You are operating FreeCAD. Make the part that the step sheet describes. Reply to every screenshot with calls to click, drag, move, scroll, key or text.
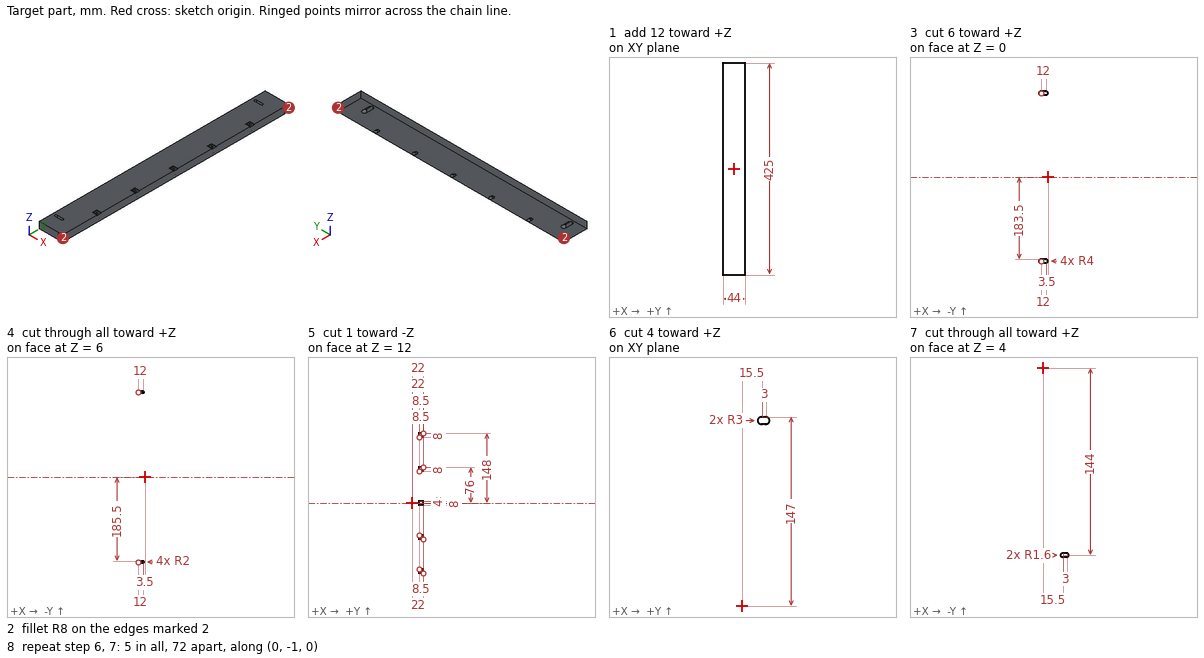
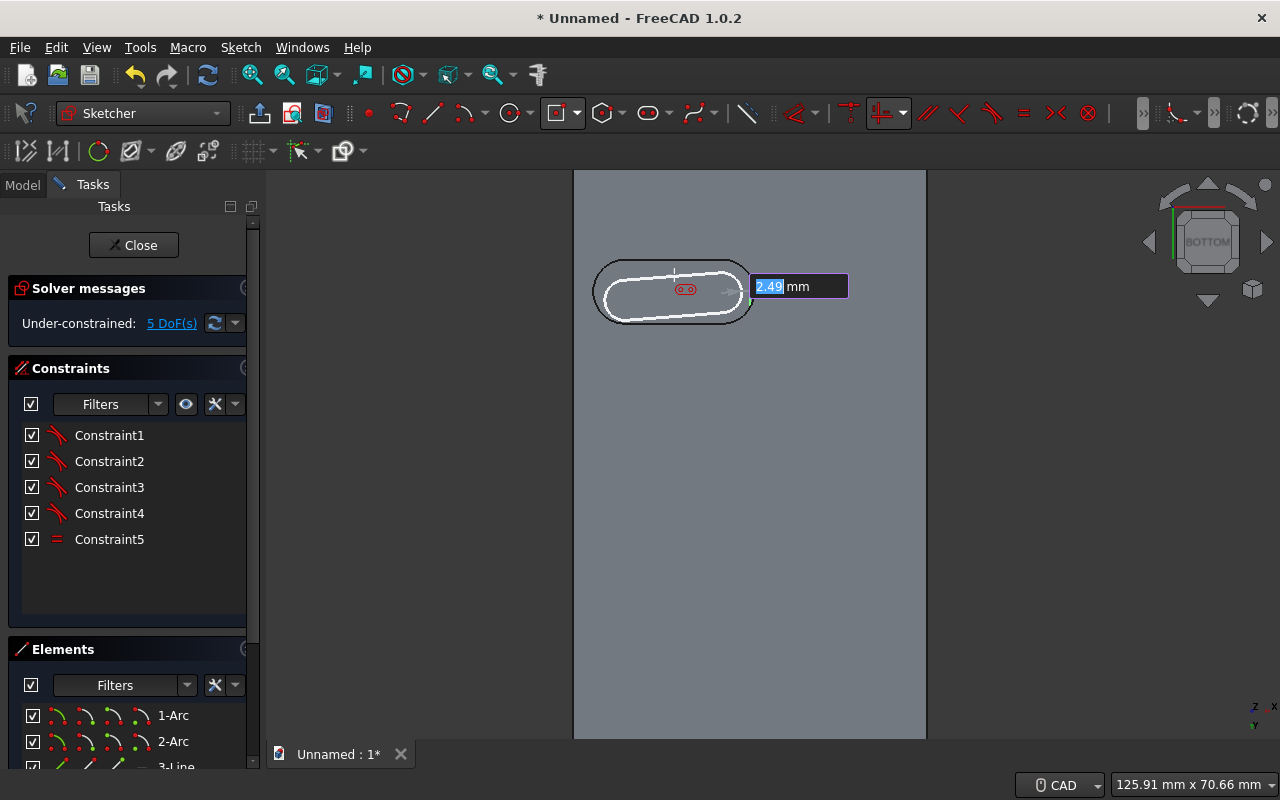
click(674, 276)
key(Escape)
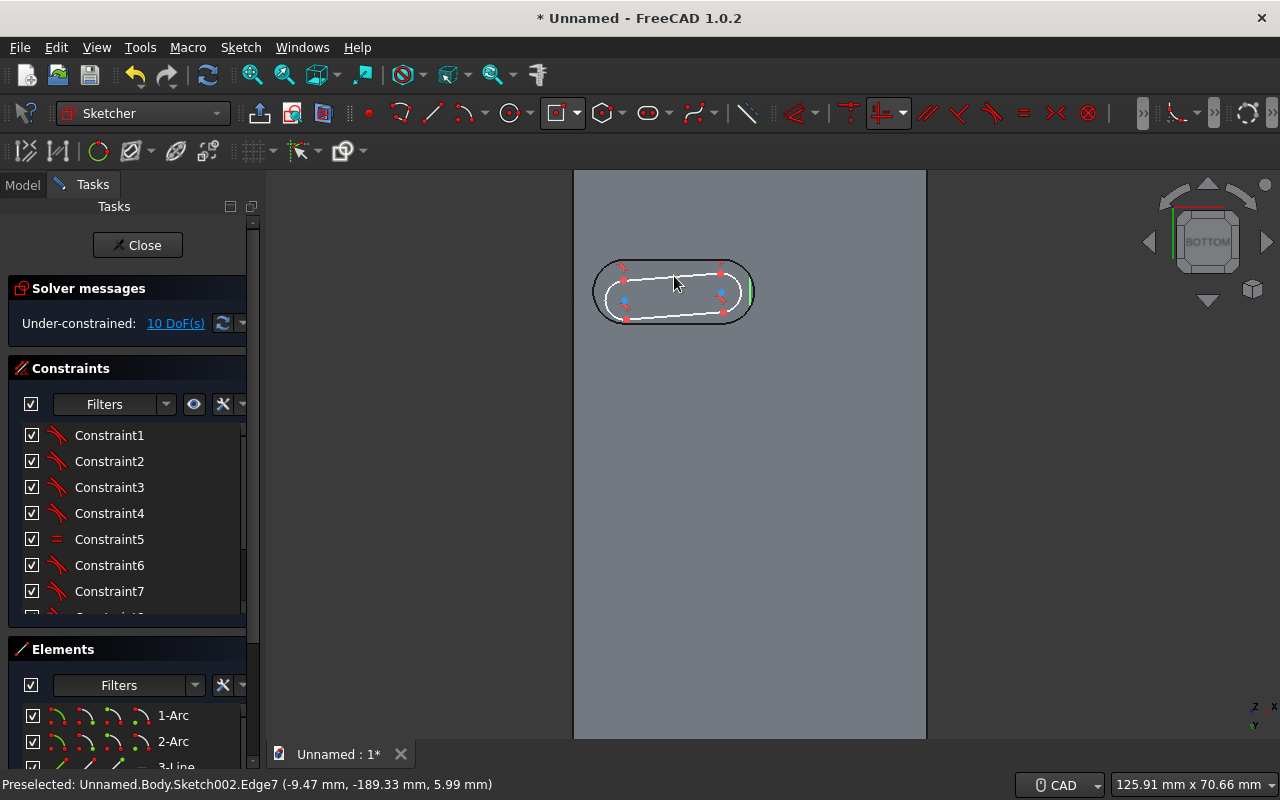
scroll(708, 287, down, 11)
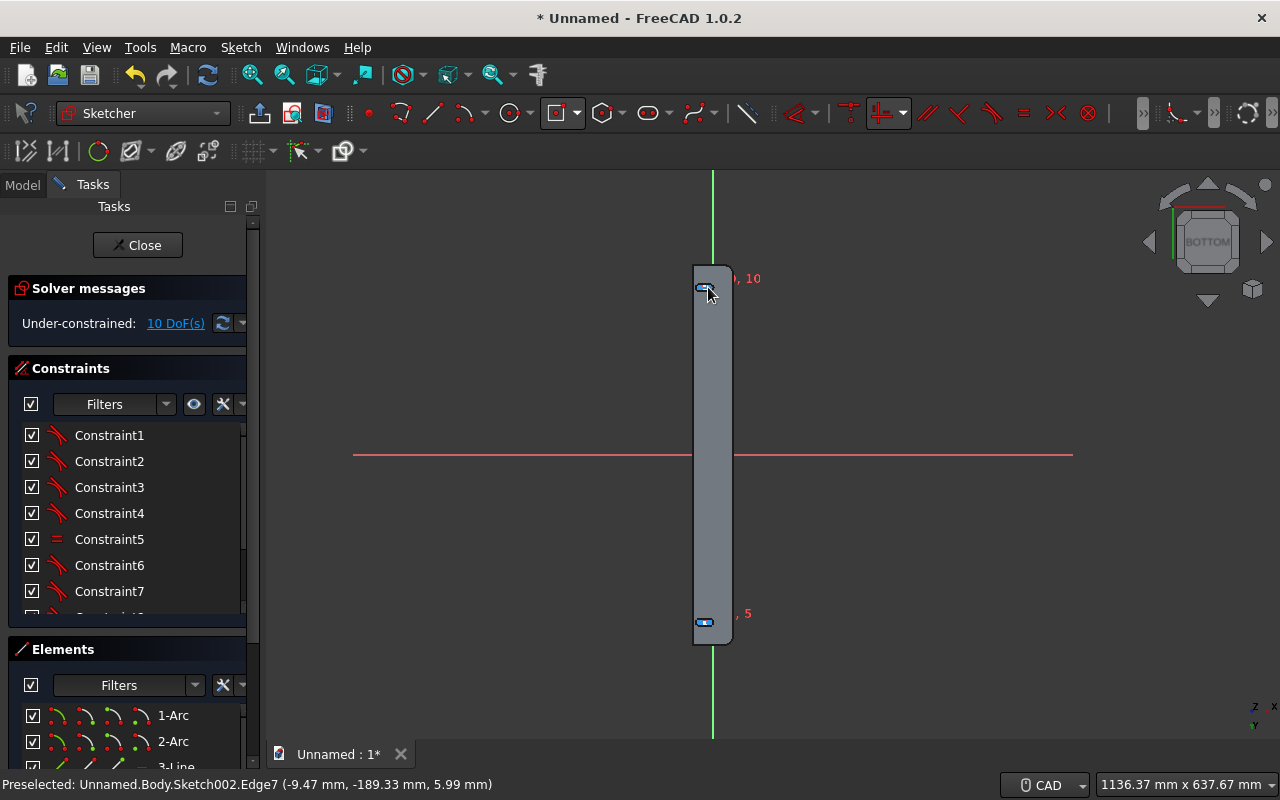
scroll(702, 622, up, 9)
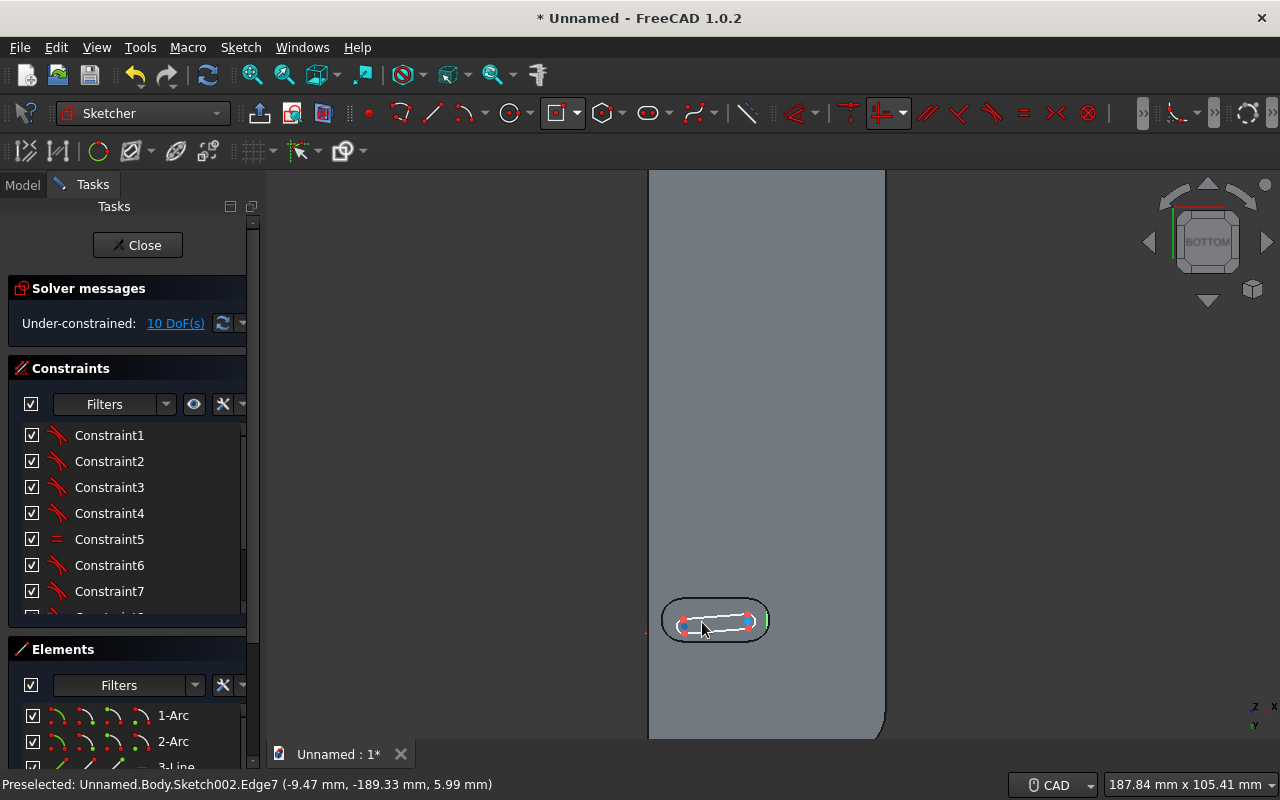
click(703, 618)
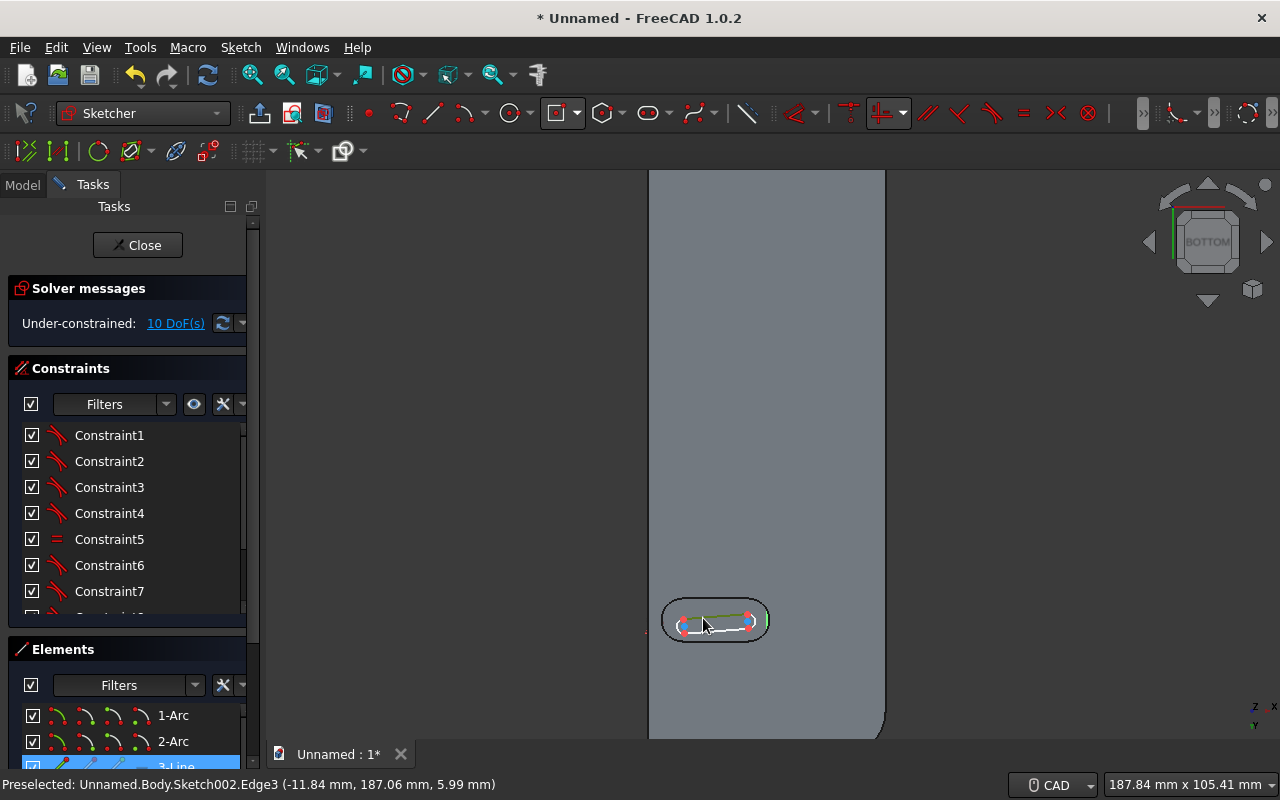
click(906, 114)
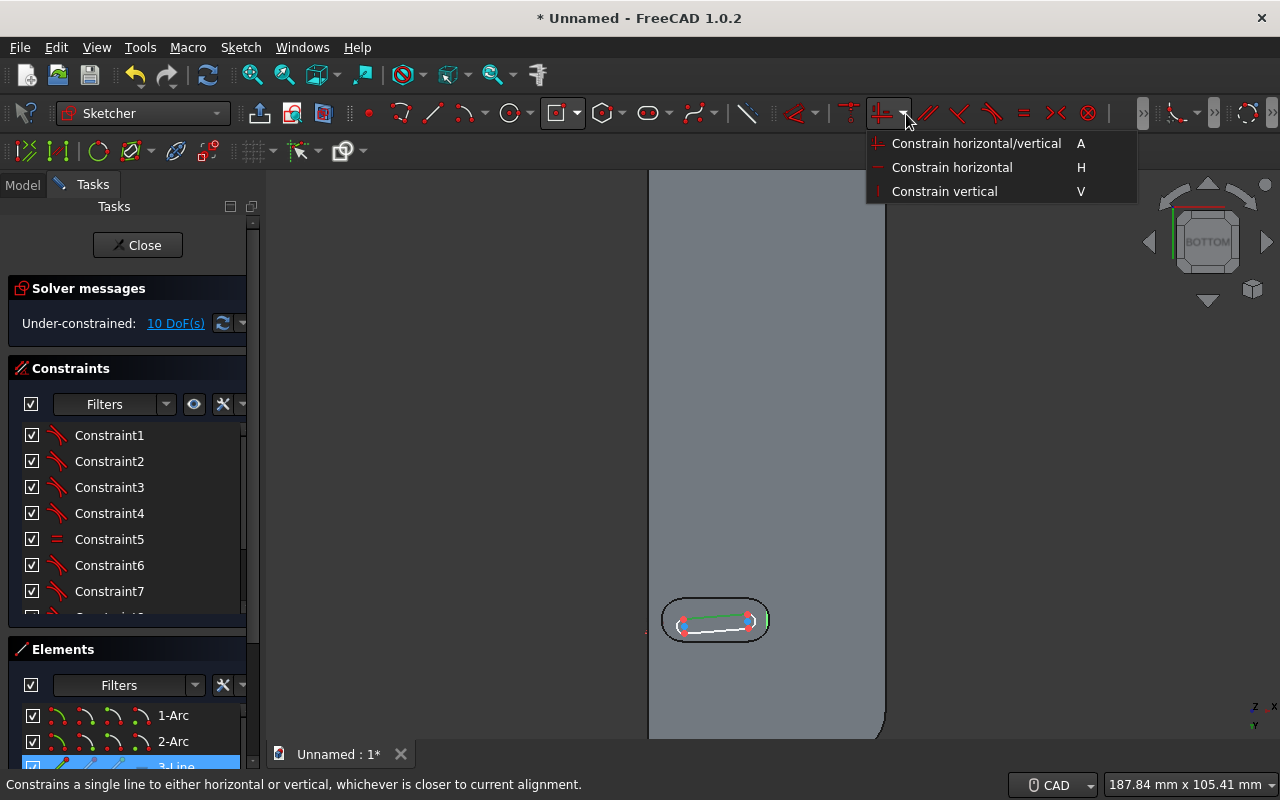
click(1002, 167)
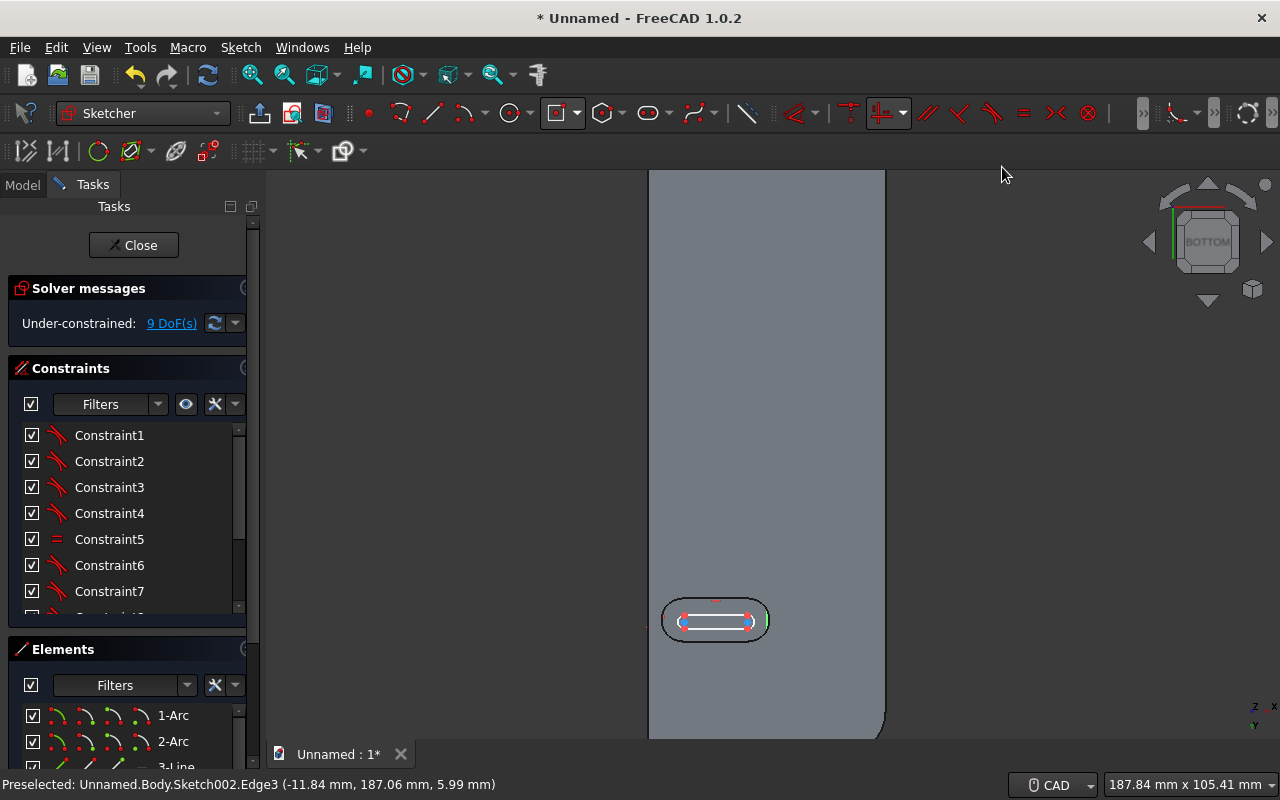
scroll(702, 622, down, 9)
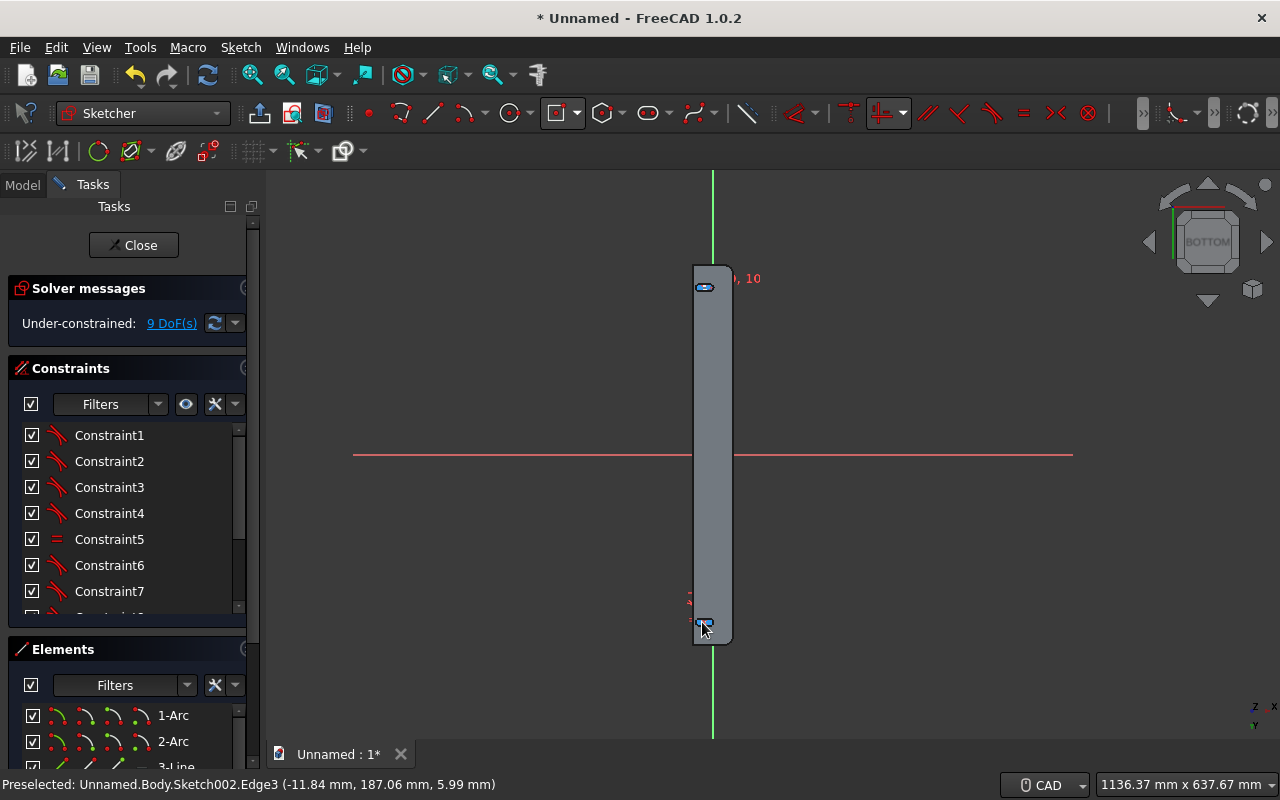
scroll(702, 286, up, 8)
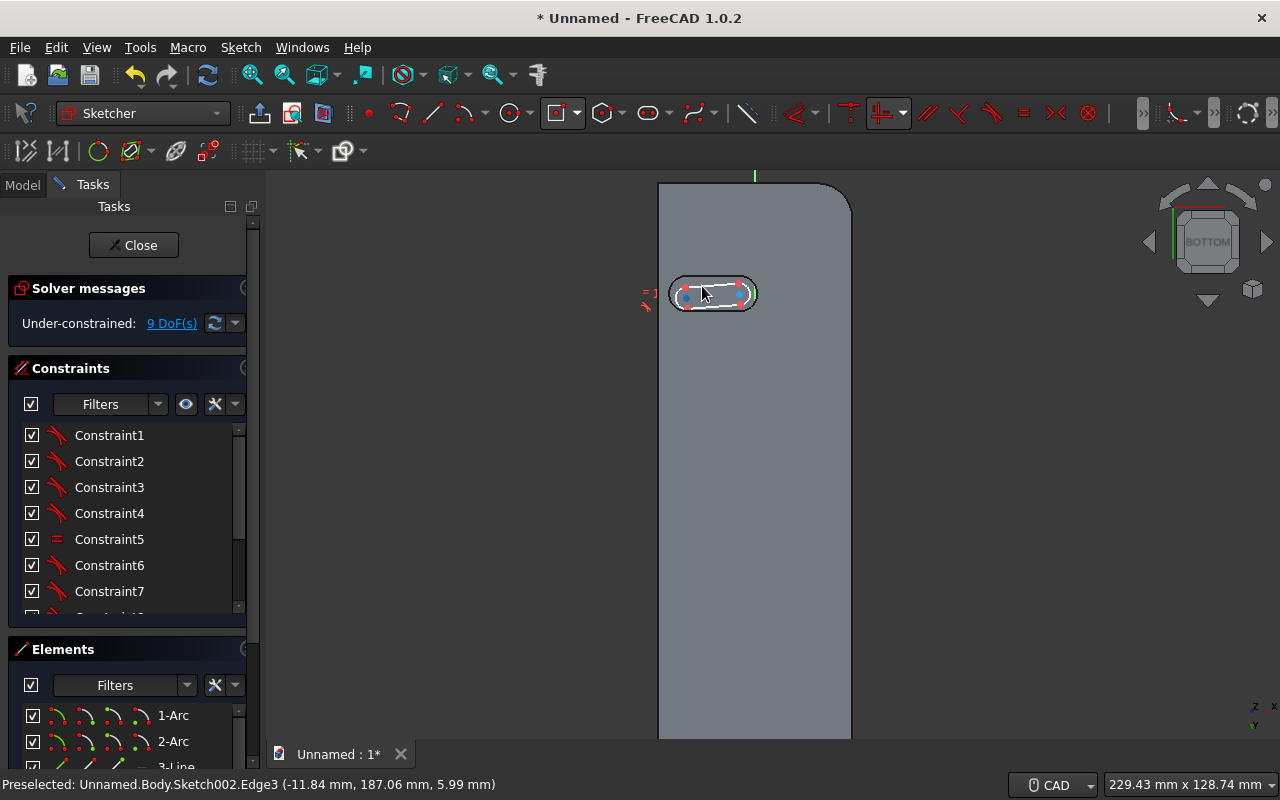
click(701, 286)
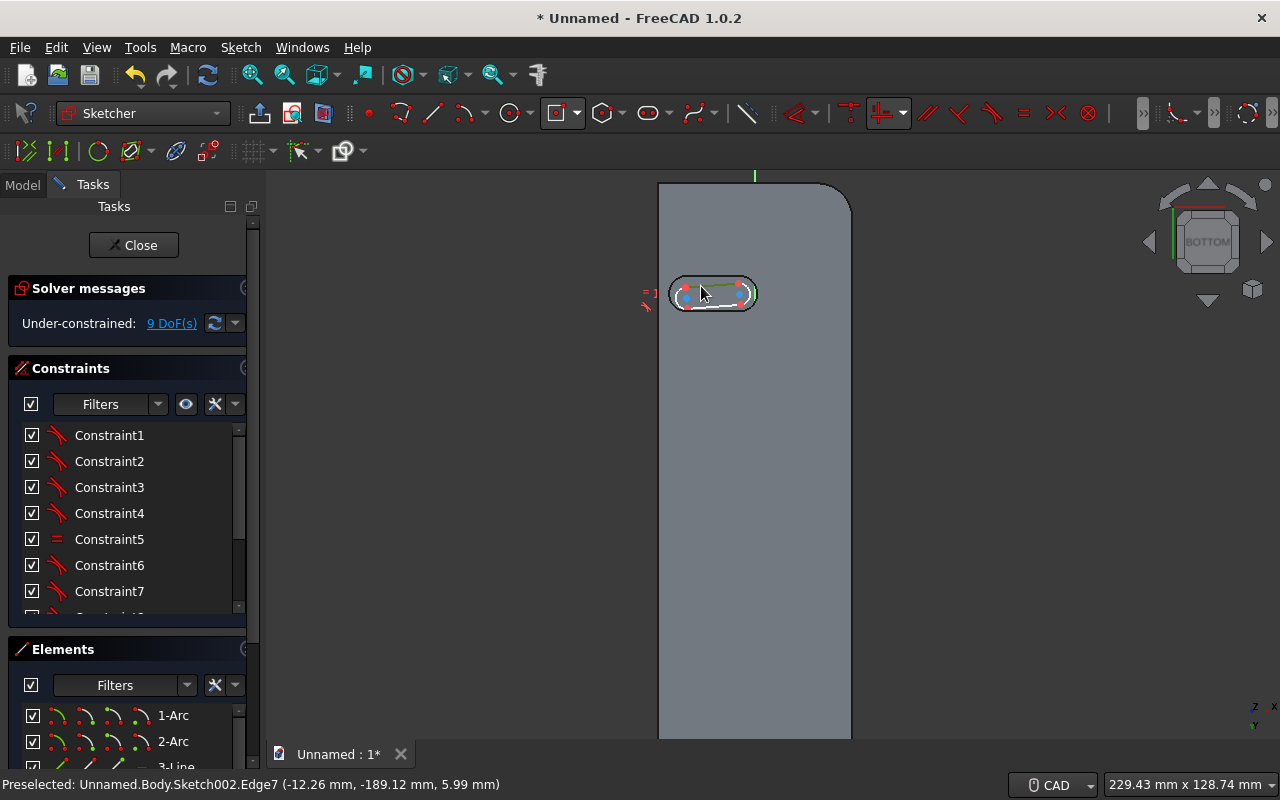
key(h)